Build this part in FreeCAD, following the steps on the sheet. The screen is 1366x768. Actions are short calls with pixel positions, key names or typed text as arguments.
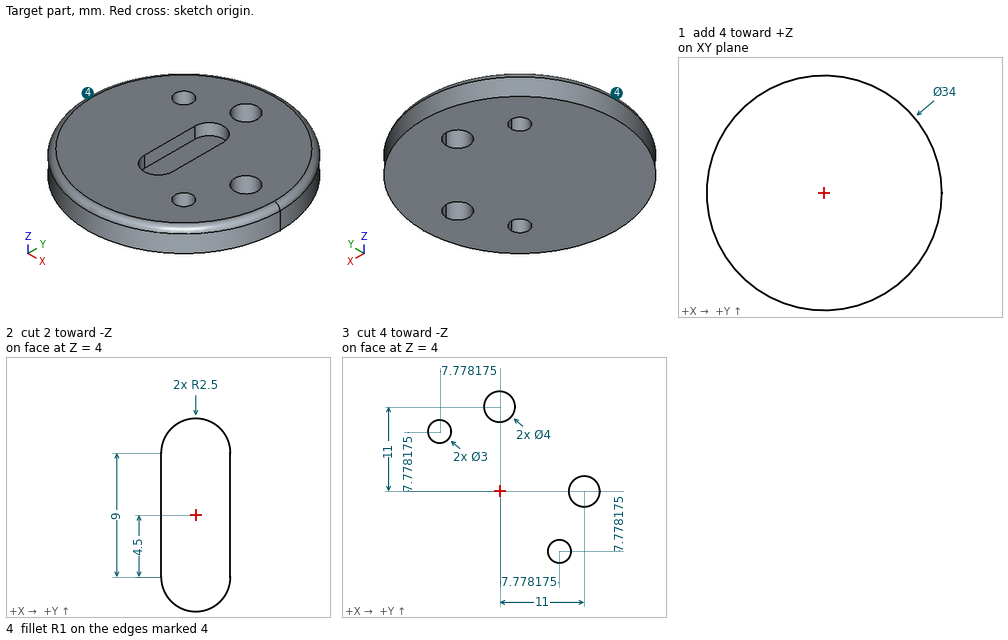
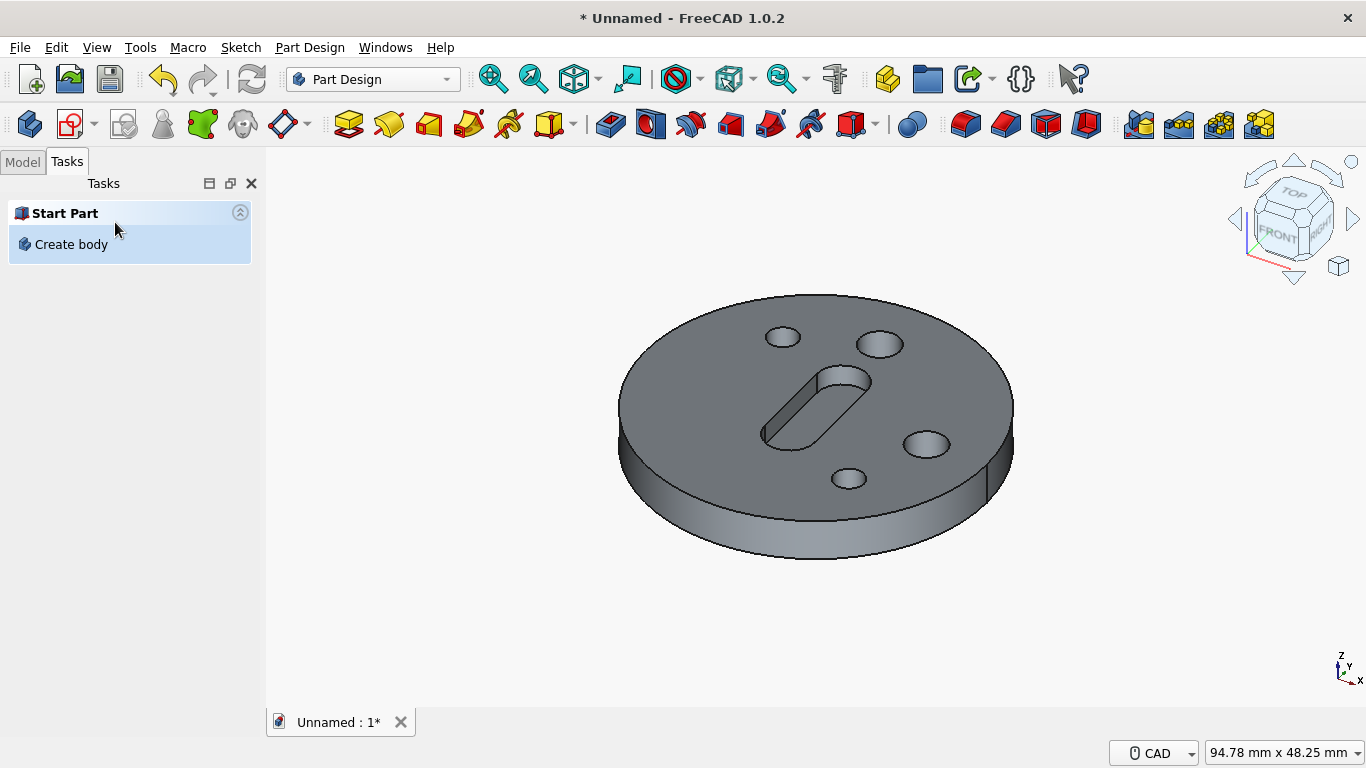
click(620, 419)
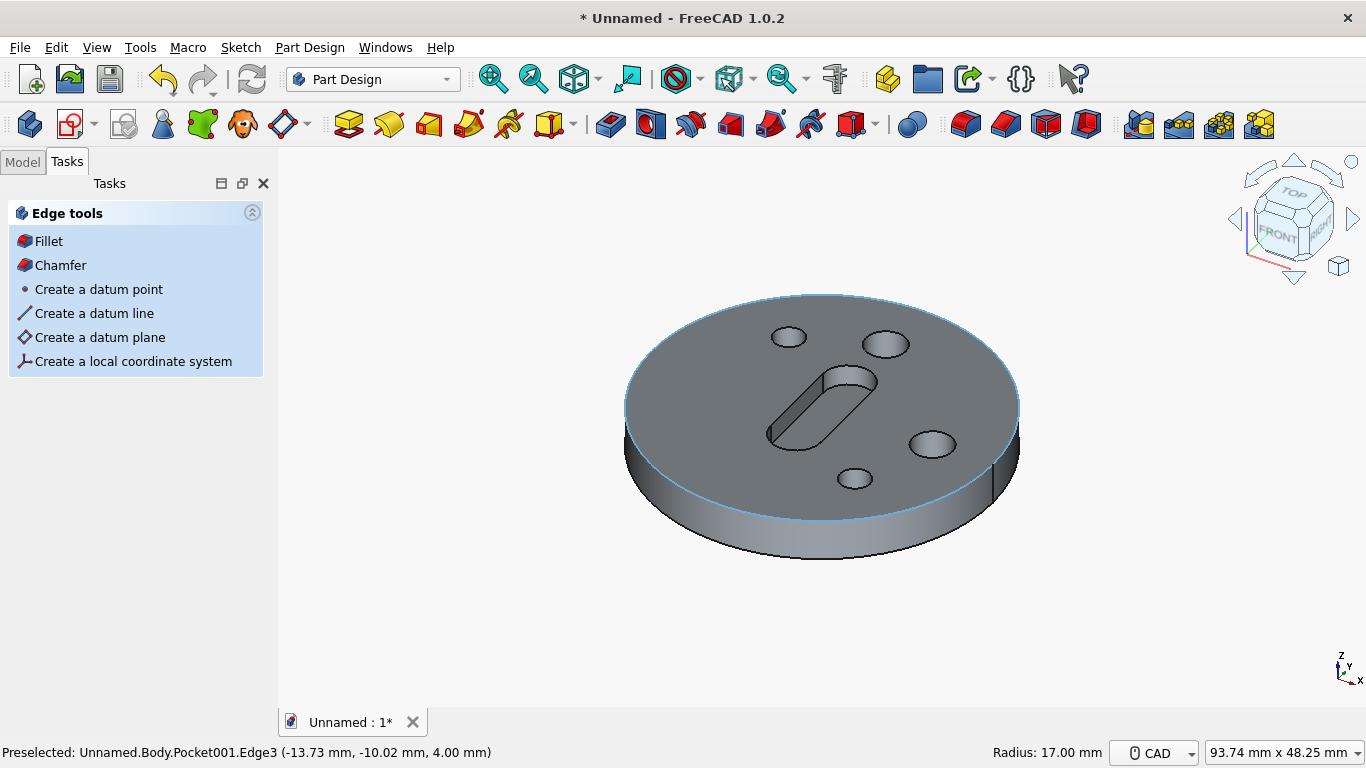
click(966, 124)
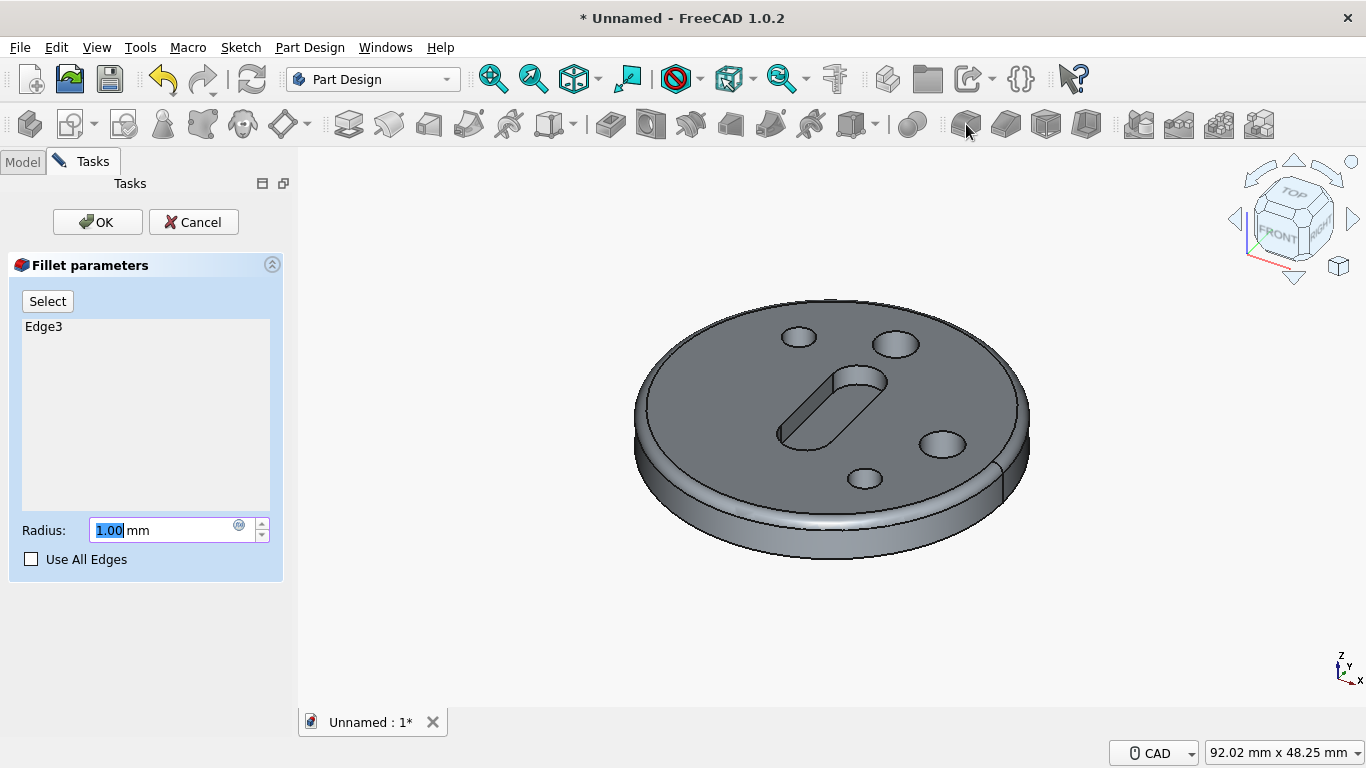
text(1)
key(Tab)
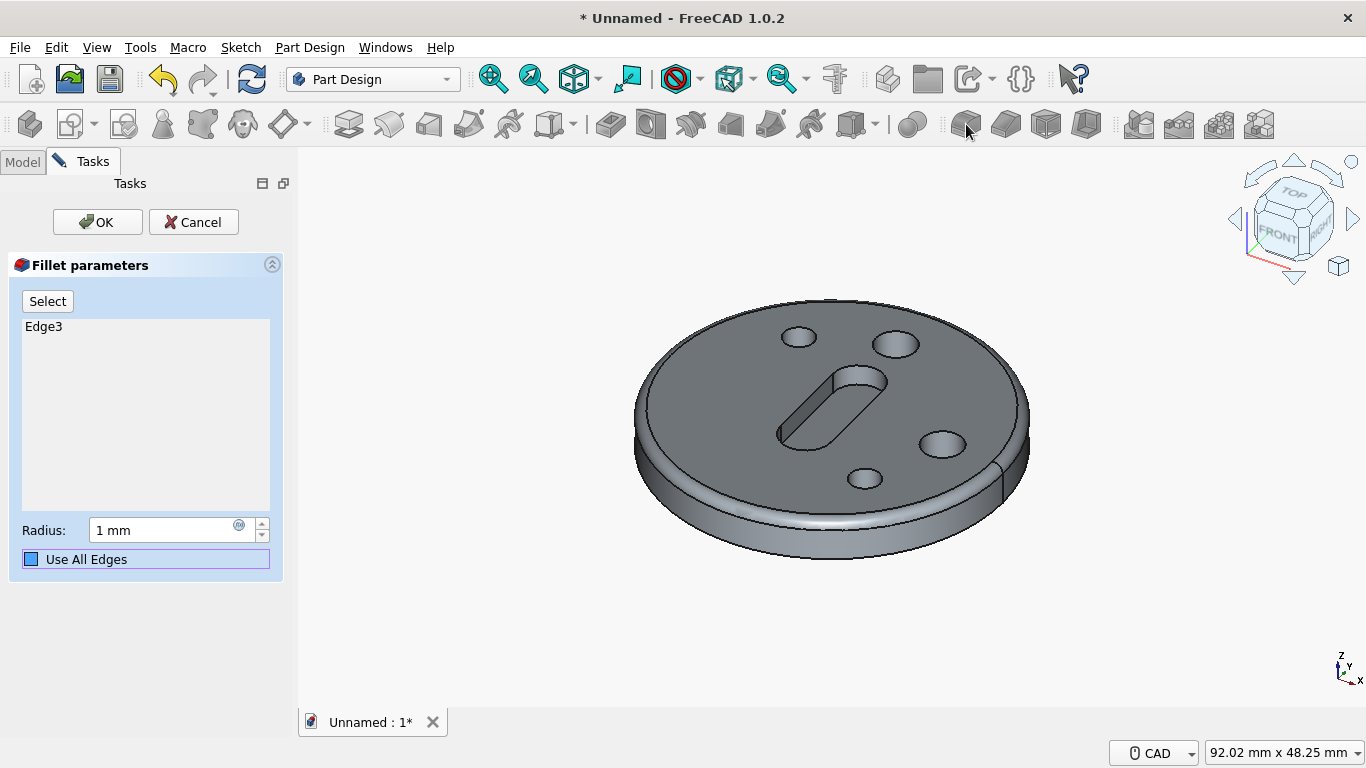
click(98, 222)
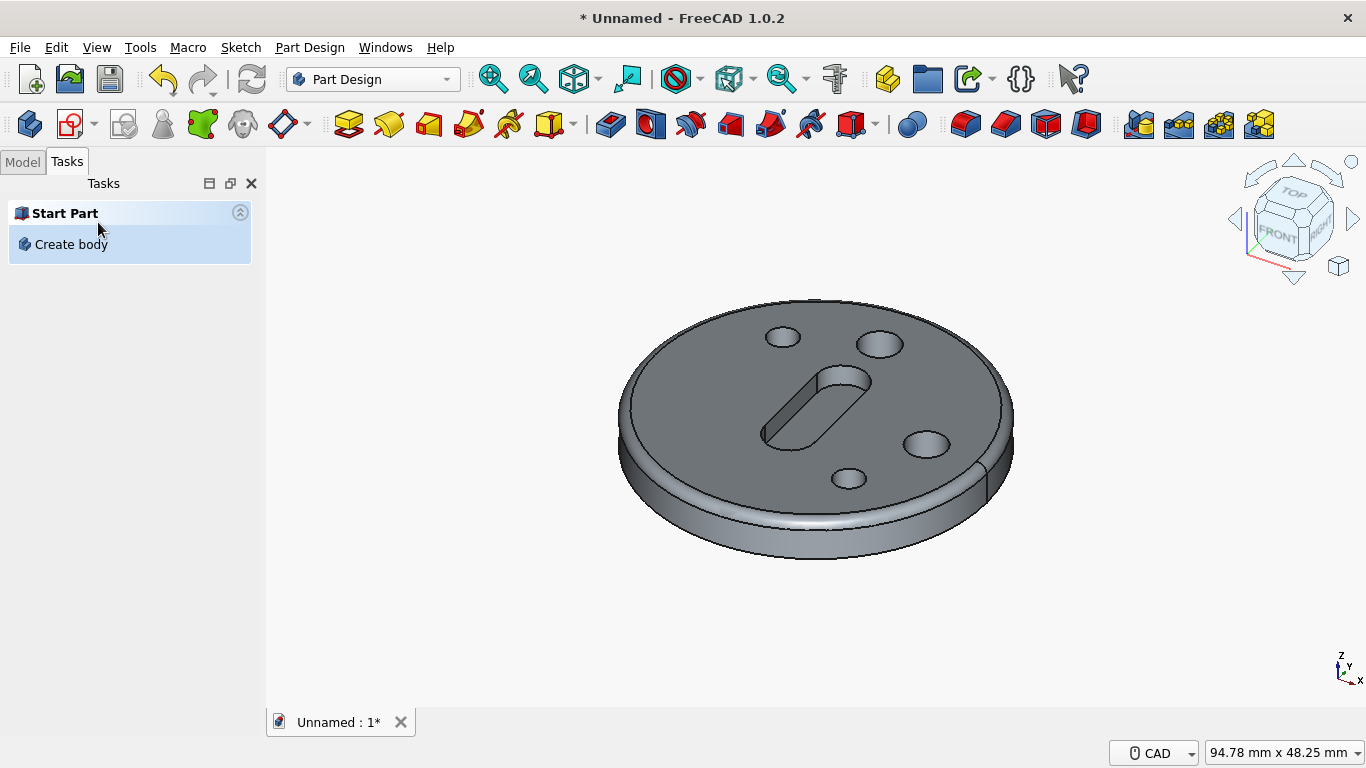
key(0)